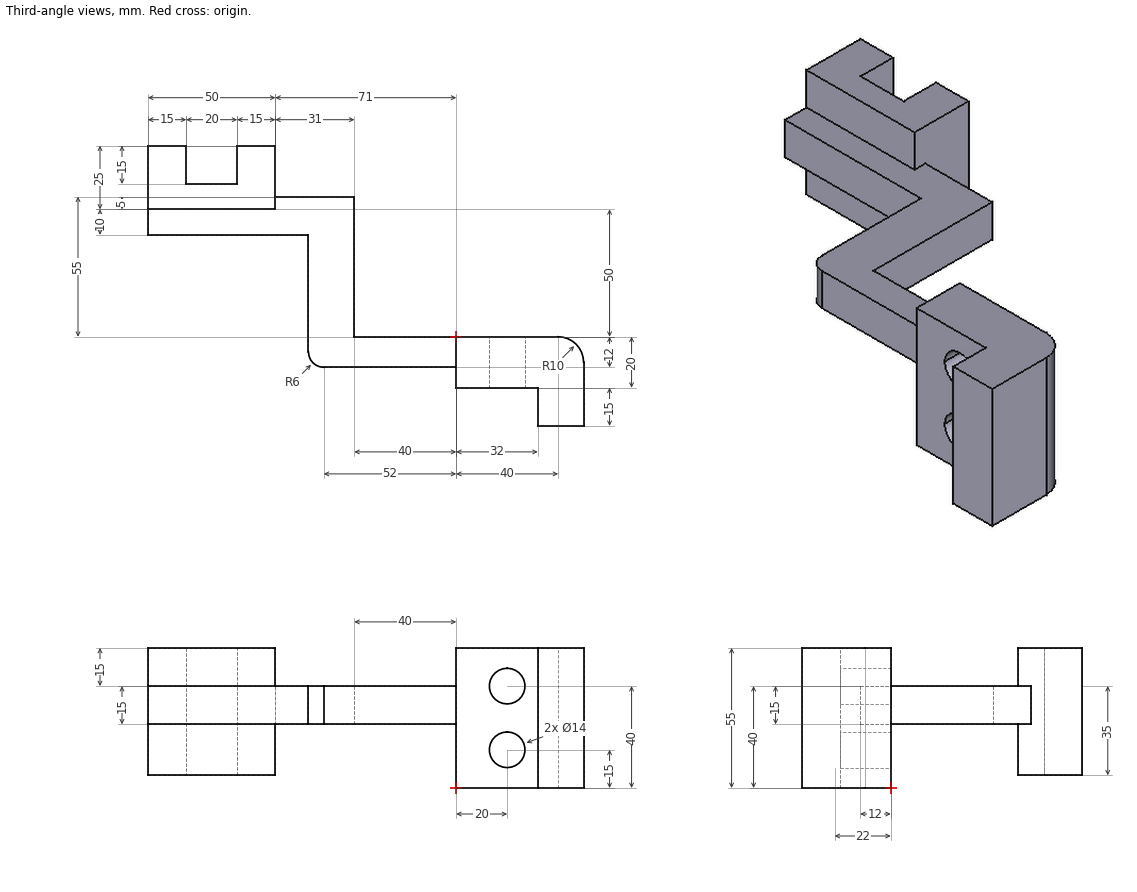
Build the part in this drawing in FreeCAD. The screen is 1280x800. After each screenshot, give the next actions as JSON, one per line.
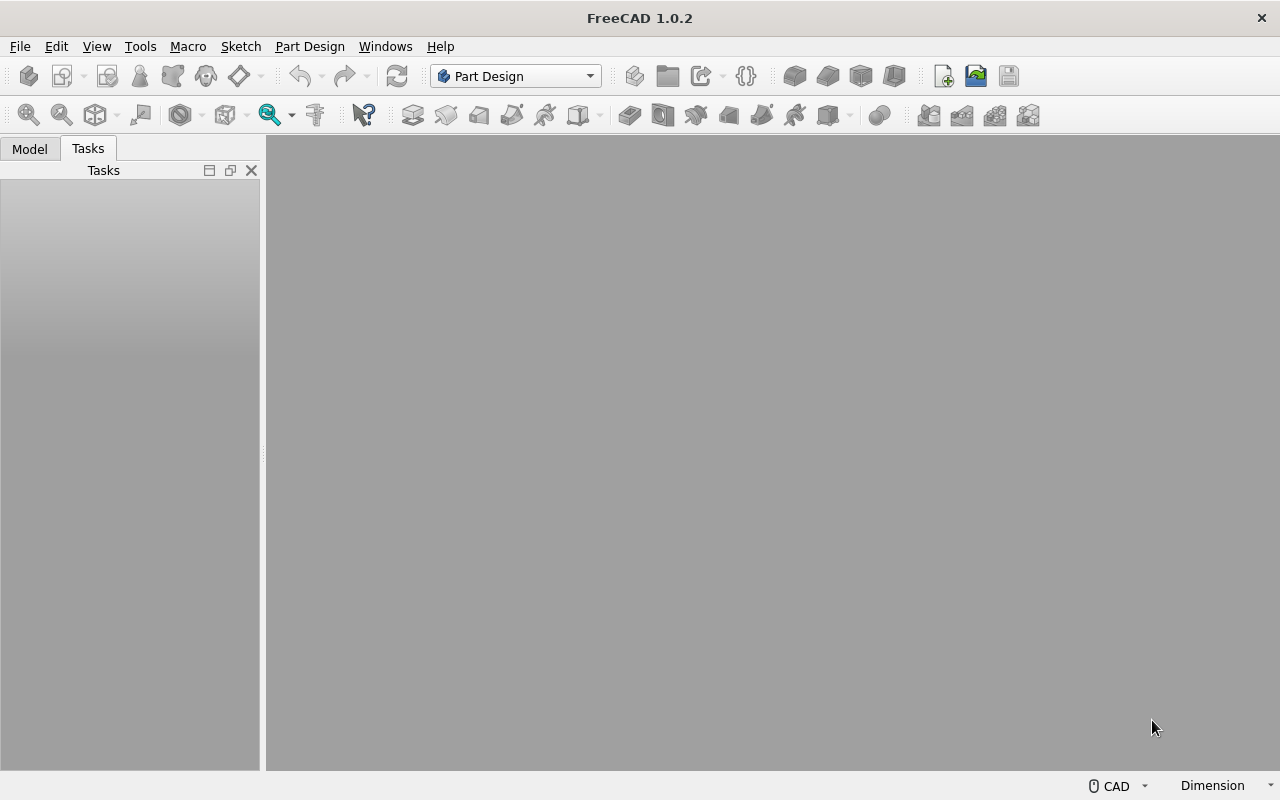
{"action": "left_click", "coordinate": [943, 76]}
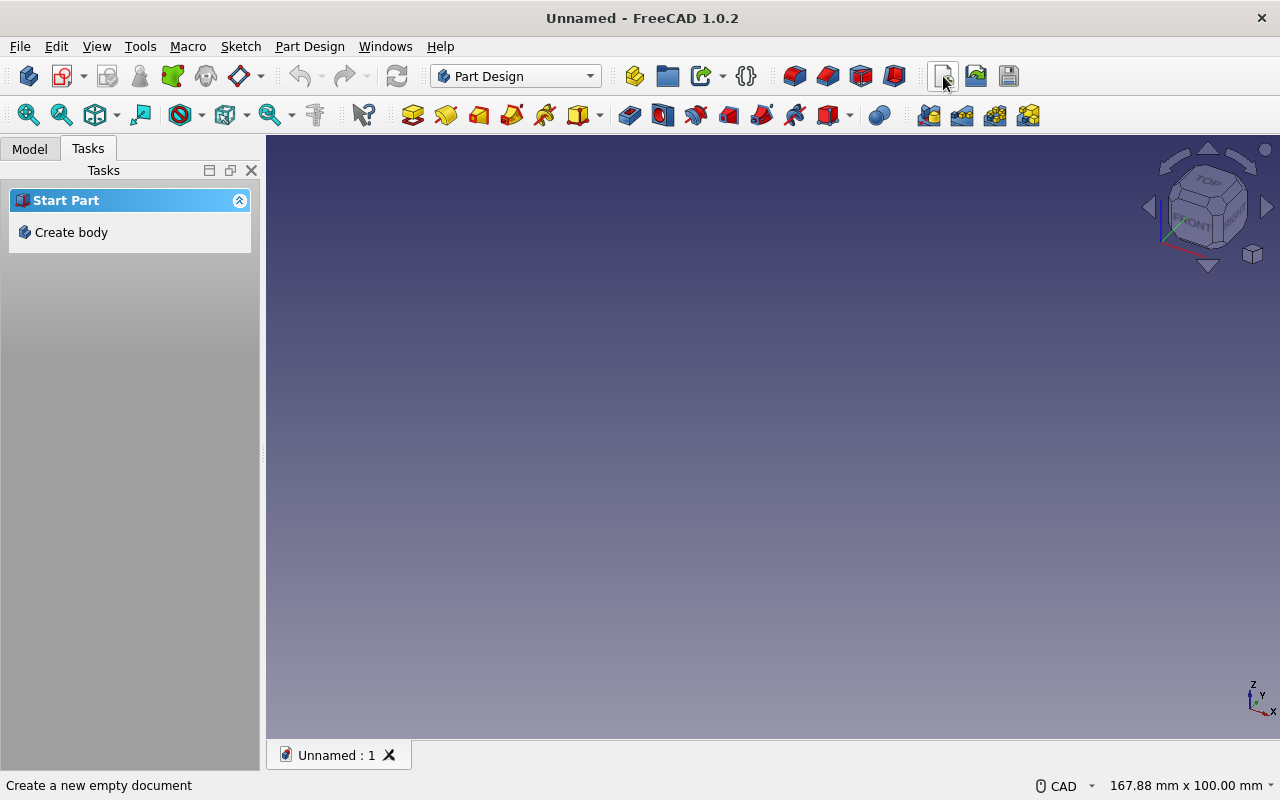
{"action": "left_click", "coordinate": [62, 76]}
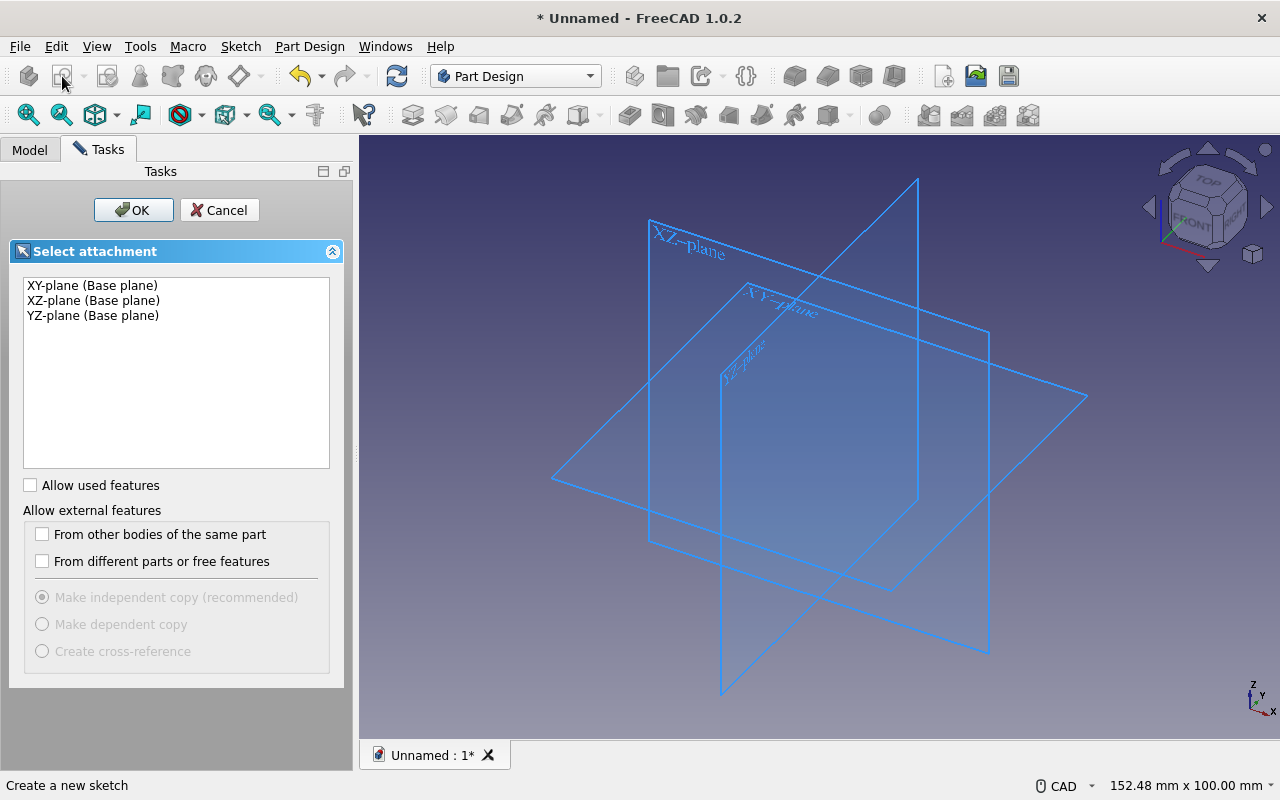
{"action": "left_click", "coordinate": [84, 286]}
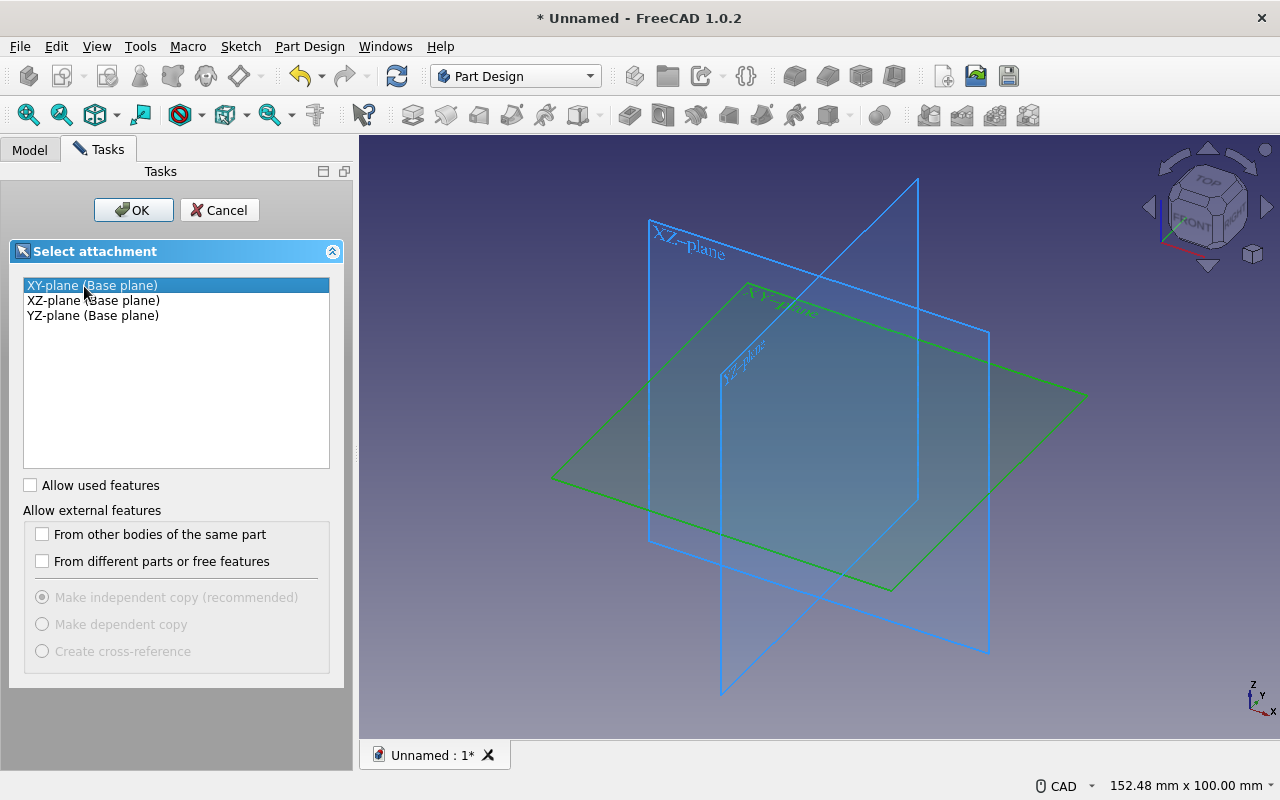
{"action": "left_click", "coordinate": [134, 210]}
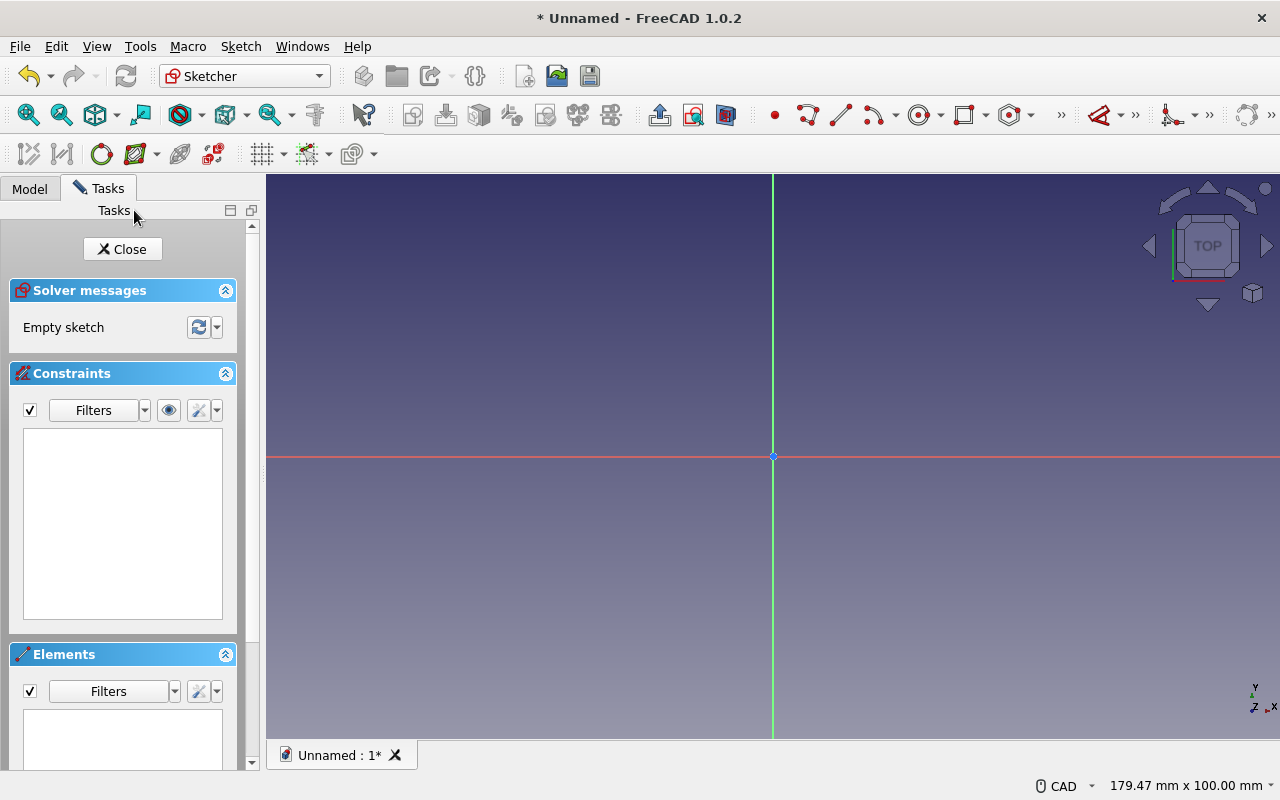
{"action": "scroll", "coordinate": [1115, 676], "scroll_direction": "up", "scroll_amount": 3}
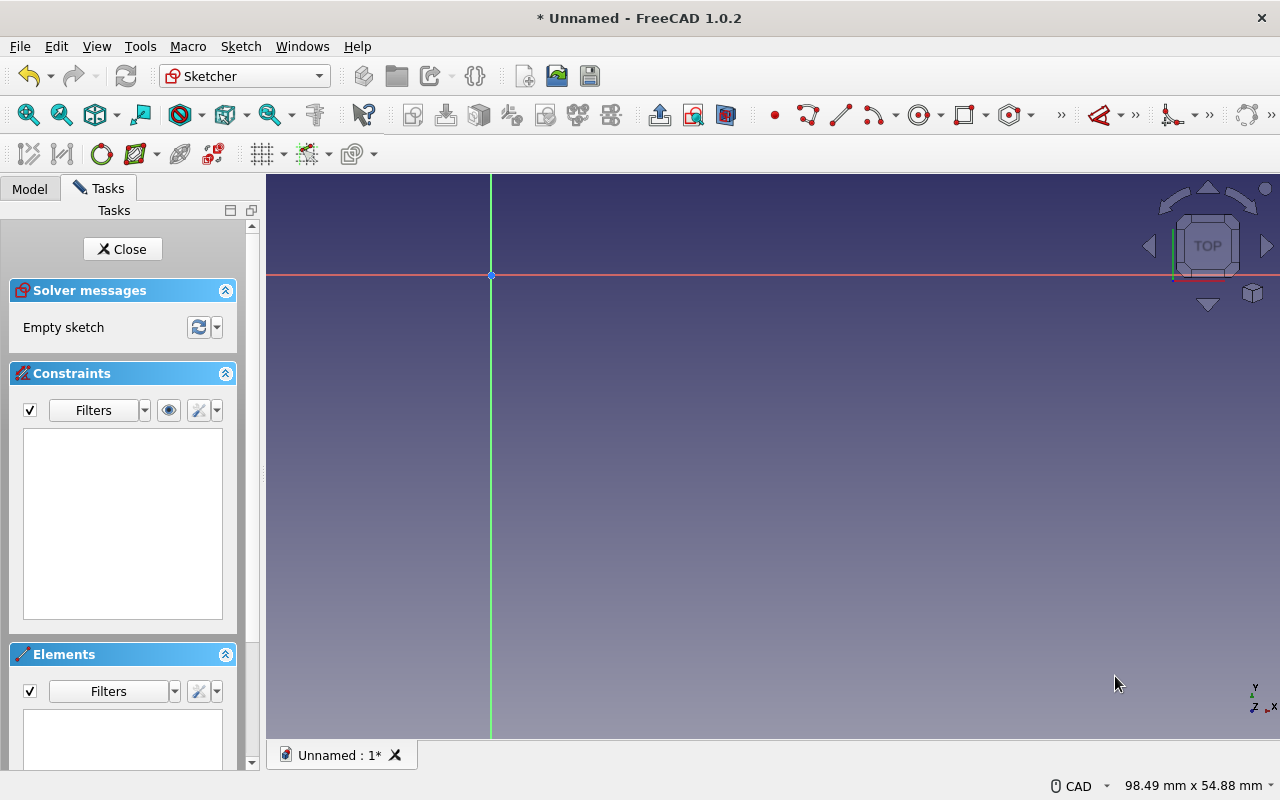
{"action": "left_click", "coordinate": [808, 116]}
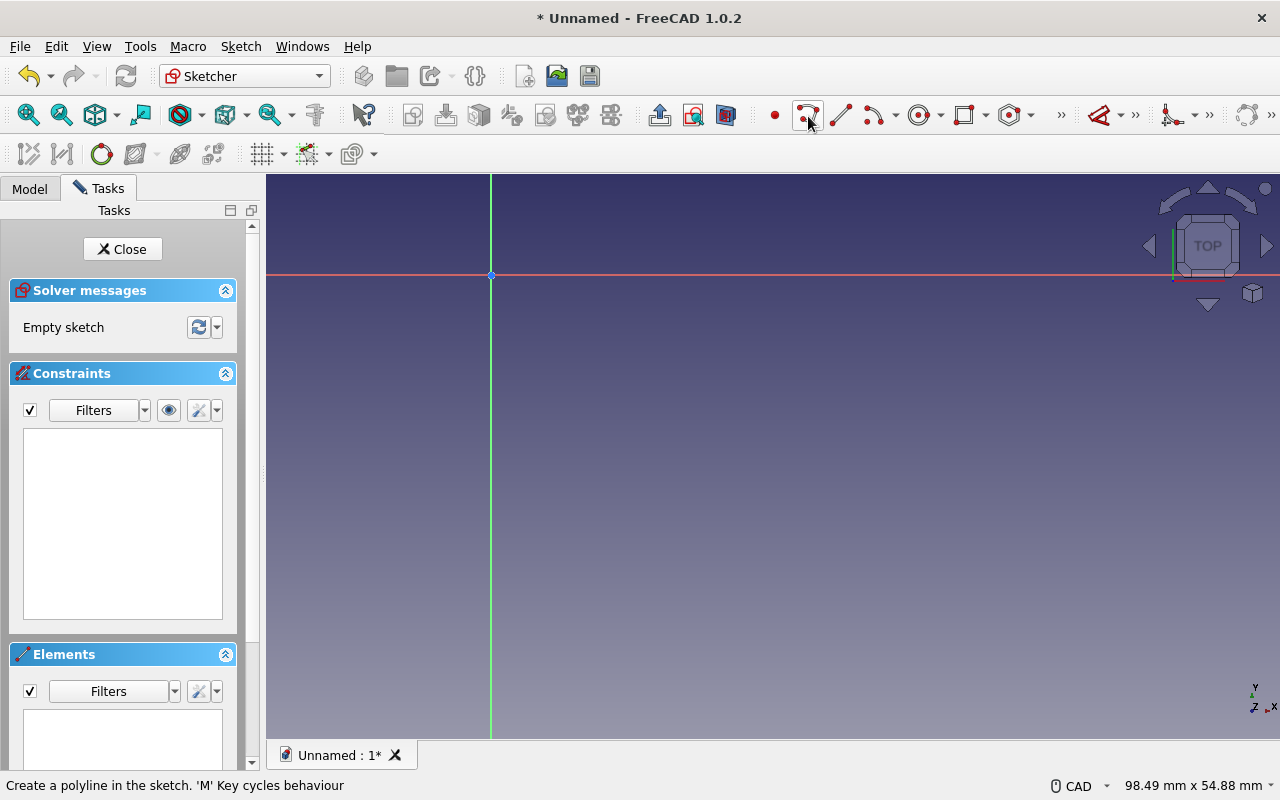
{"action": "left_click", "coordinate": [903, 275]}
{"action": "left_click", "coordinate": [491, 275]}
{"action": "left_click", "coordinate": [500, 481]}
{"action": "left_click", "coordinate": [821, 481]}
{"action": "left_click", "coordinate": [821, 636]}
{"action": "left_click", "coordinate": [1006, 636]}
{"action": "left_click", "coordinate": [1006, 378]}
{"action": "right_click", "coordinate": [1006, 378]}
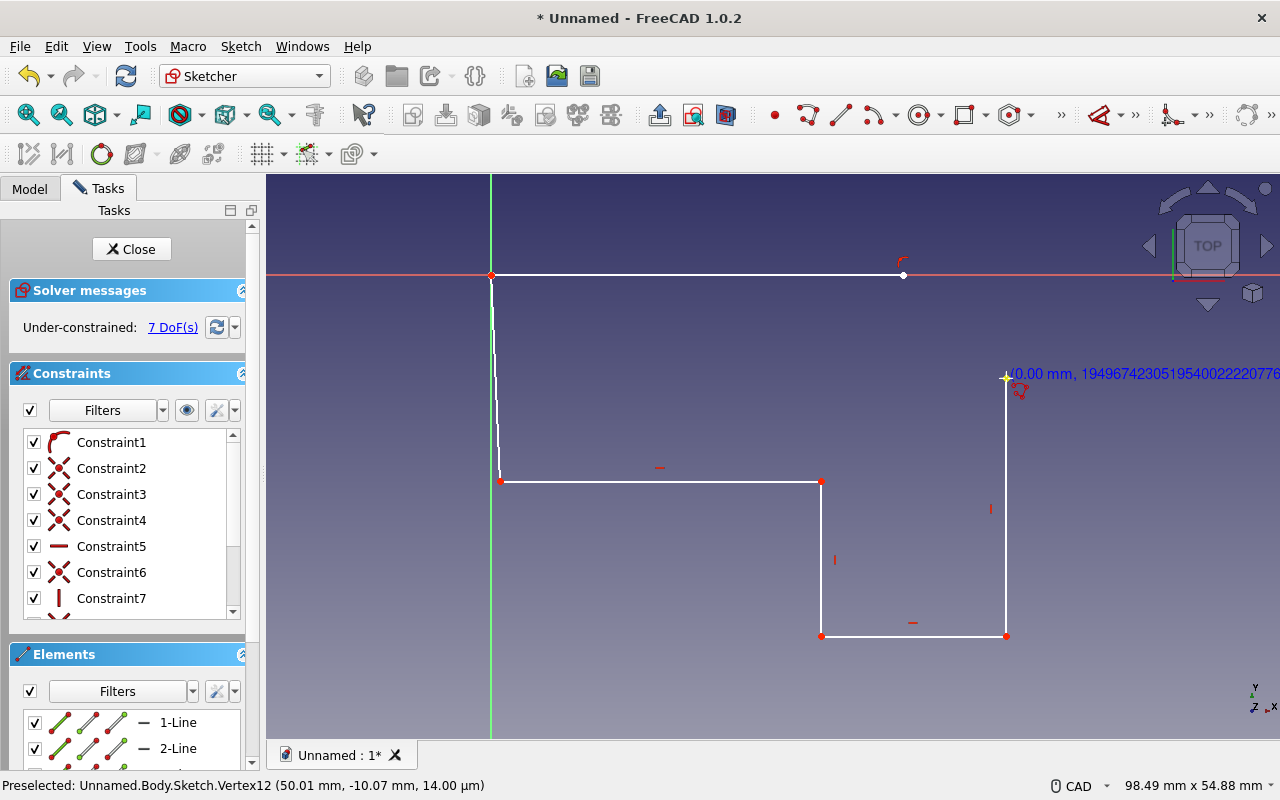
{"action": "left_click", "coordinate": [896, 116]}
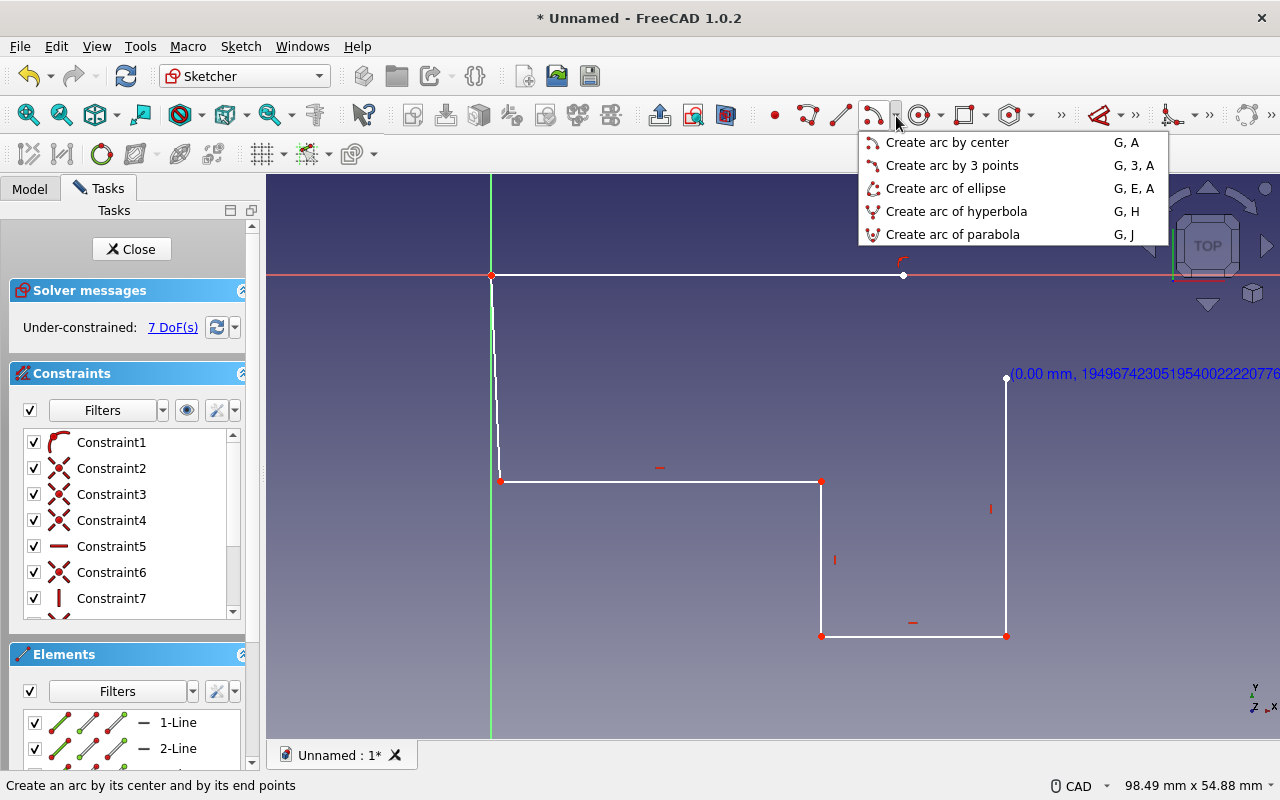
{"action": "left_click", "coordinate": [1014, 166]}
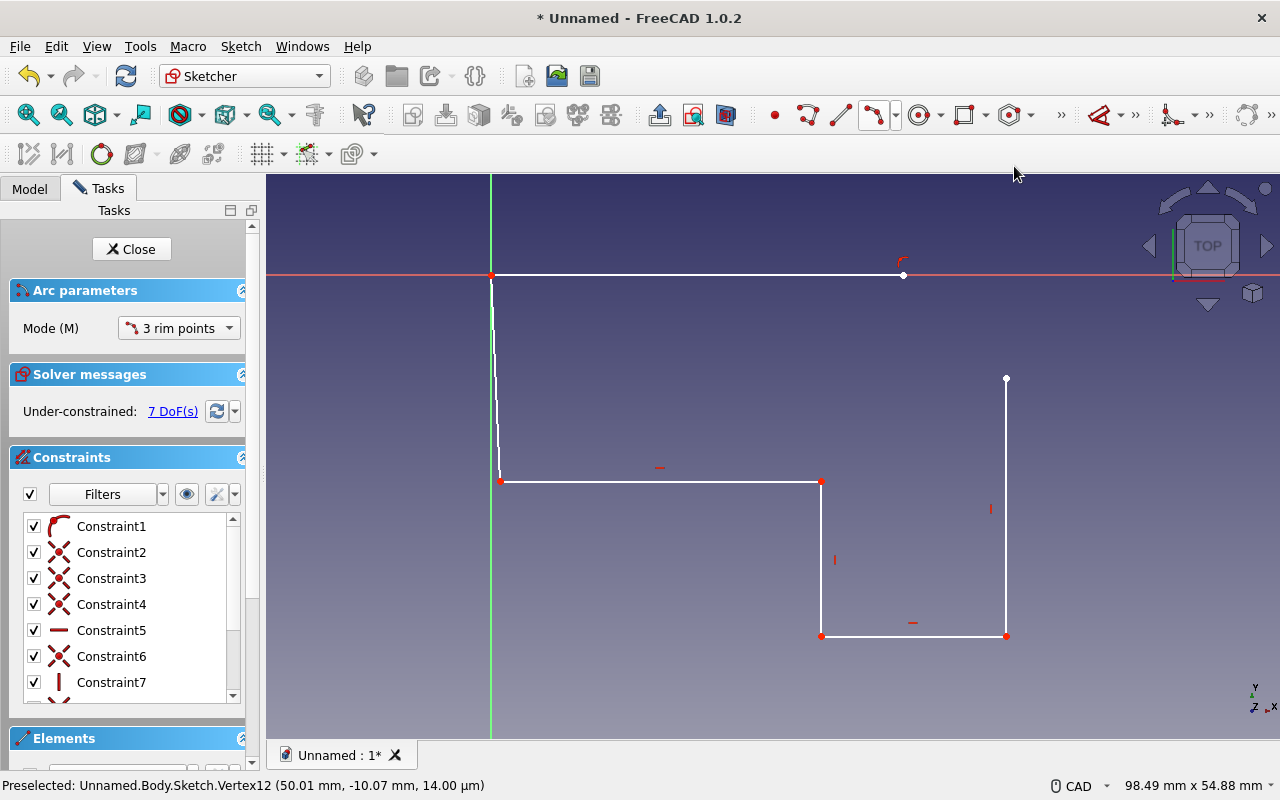
{"action": "left_click", "coordinate": [1006, 379]}
{"action": "left_click", "coordinate": [903, 275]}
{"action": "left_click", "coordinate": [976, 305]}
{"action": "key", "text": "Escape"}